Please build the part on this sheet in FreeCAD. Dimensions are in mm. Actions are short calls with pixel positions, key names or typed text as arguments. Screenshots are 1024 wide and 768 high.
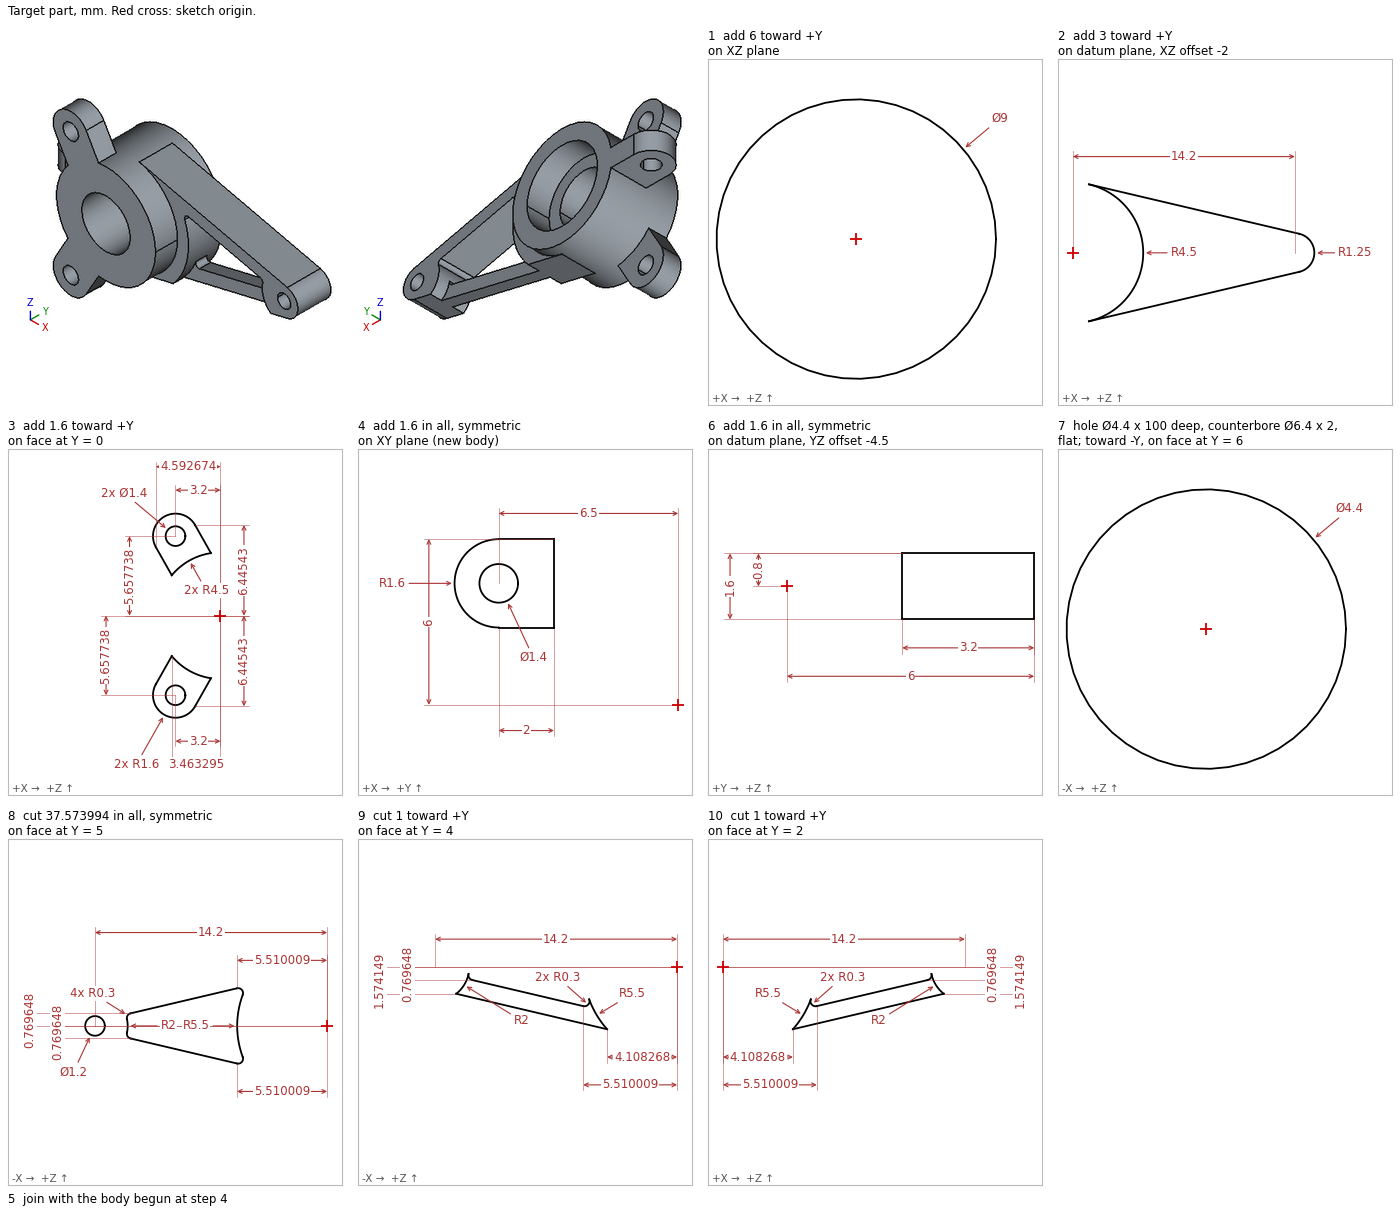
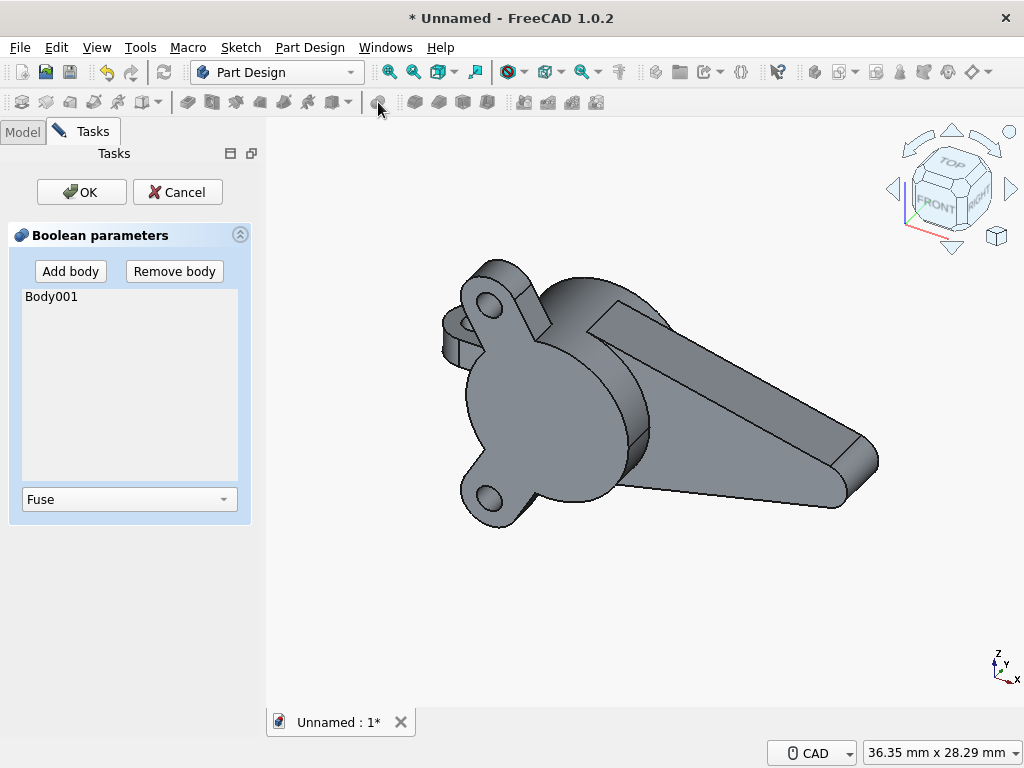
click(82, 192)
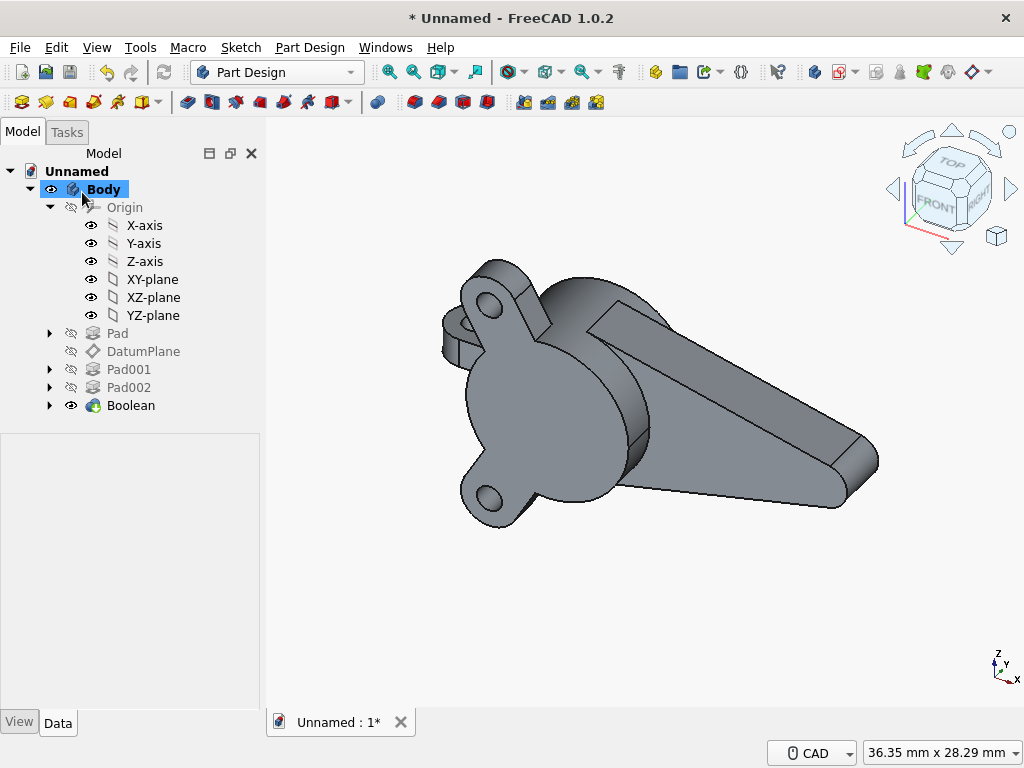
click(136, 315)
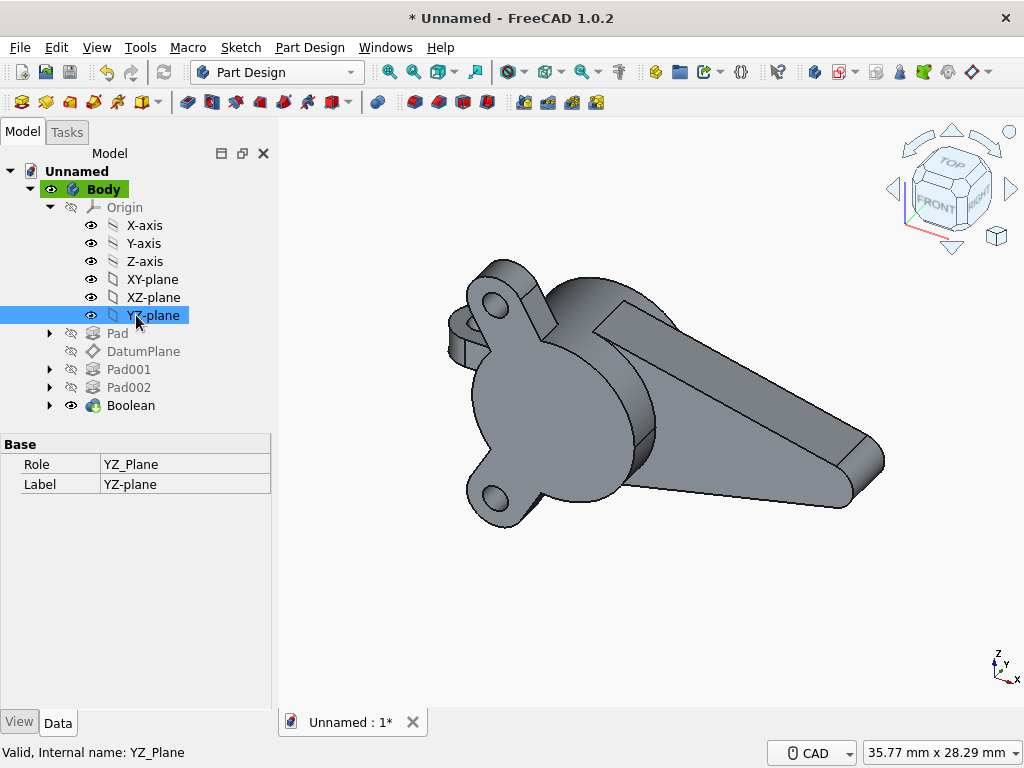
click(972, 72)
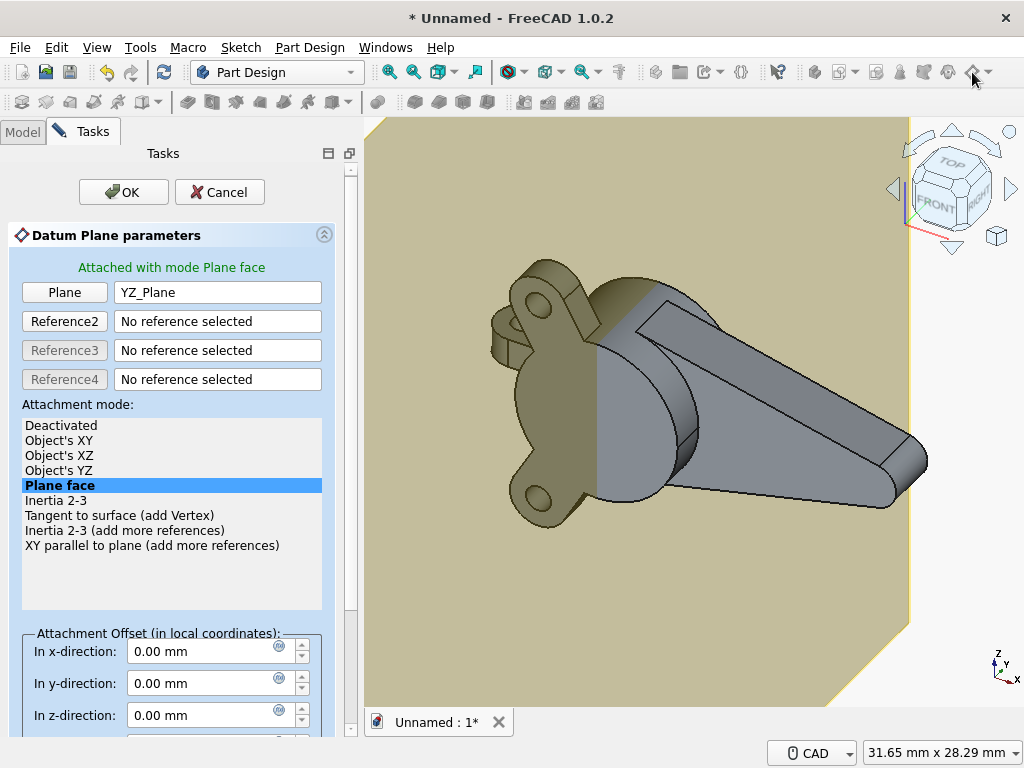
triple_click(210, 715)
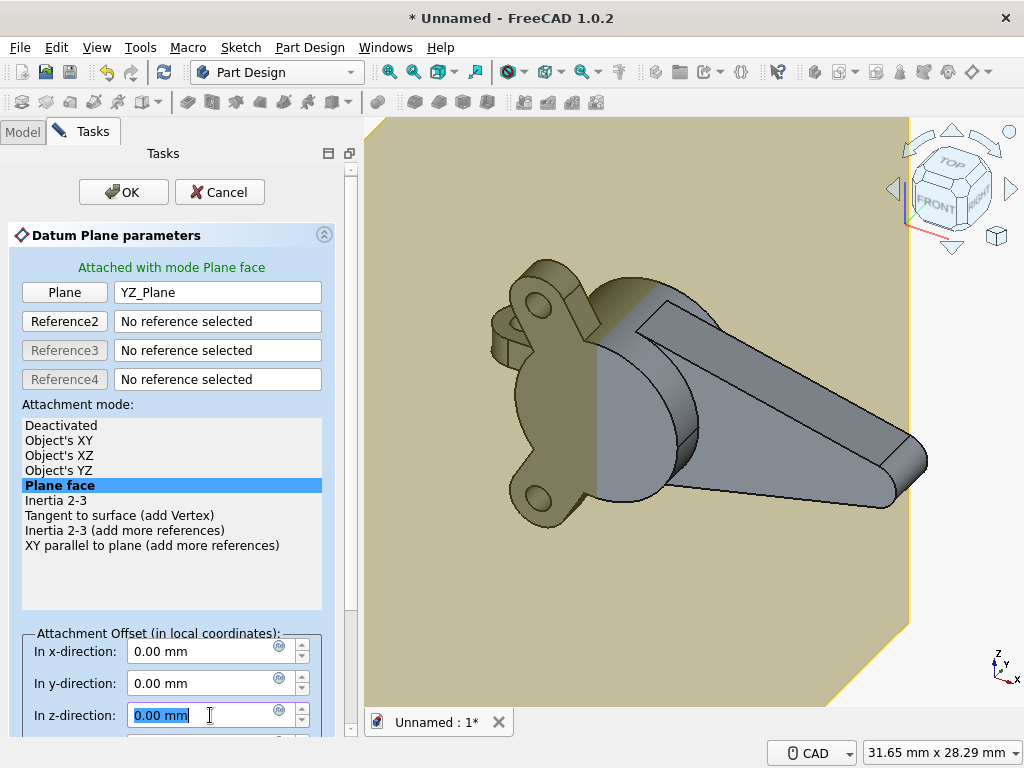
text(-4.5)
key(Tab)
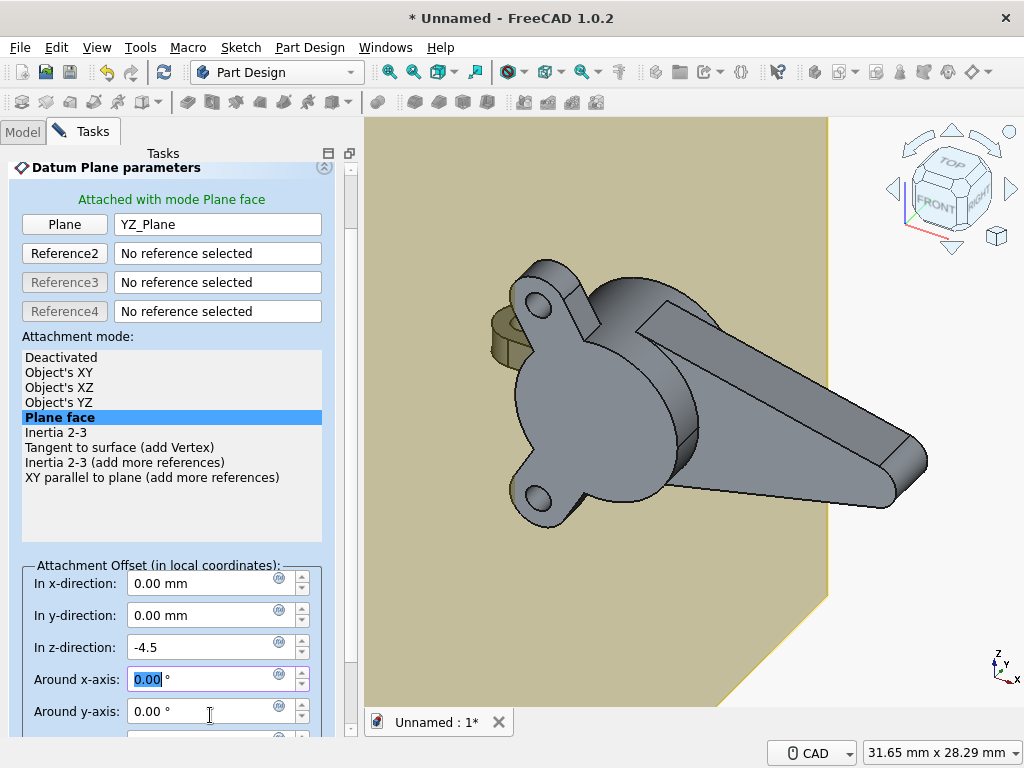
scroll(351, 450, up, 2)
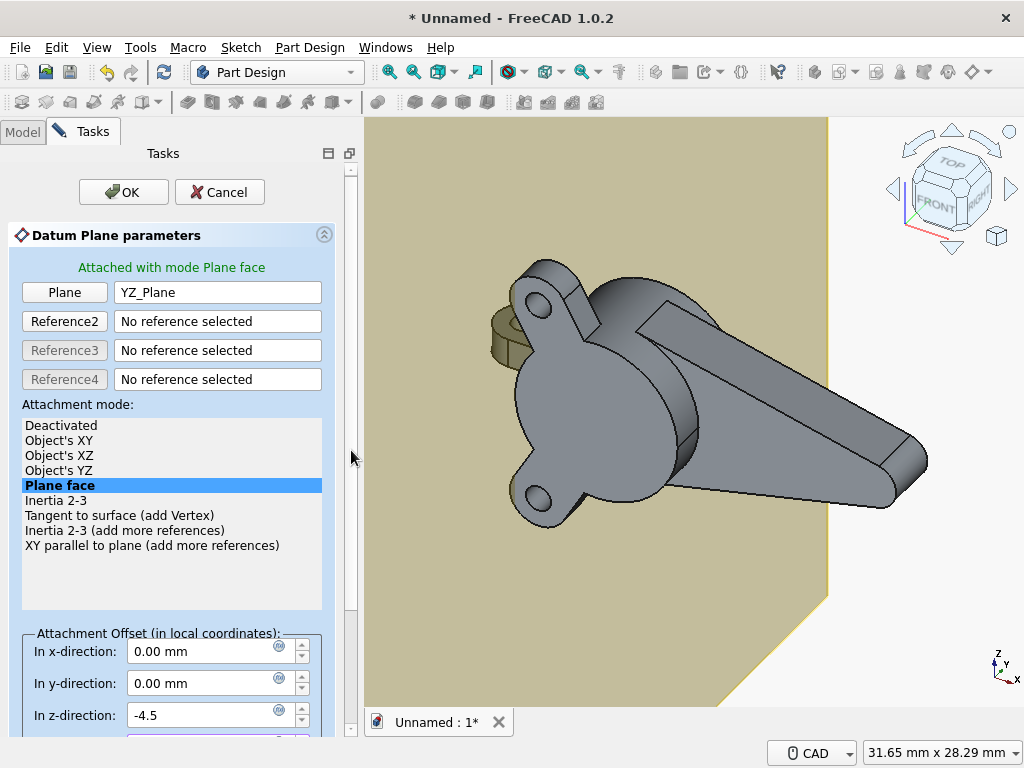
click(124, 192)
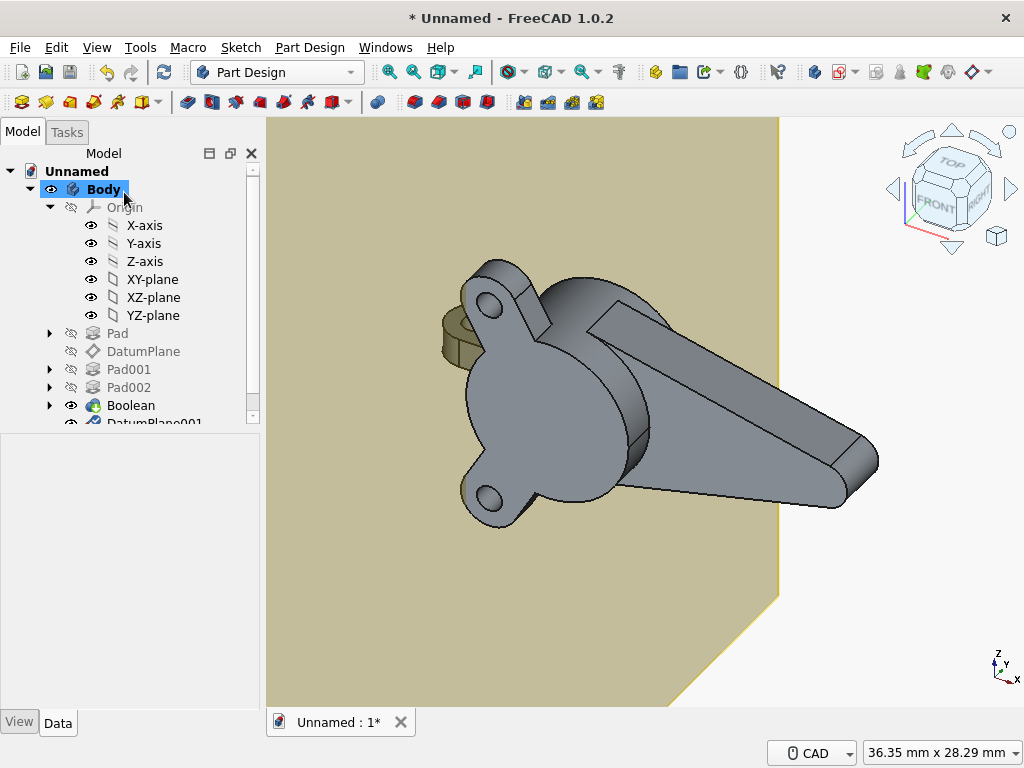
click(116, 423)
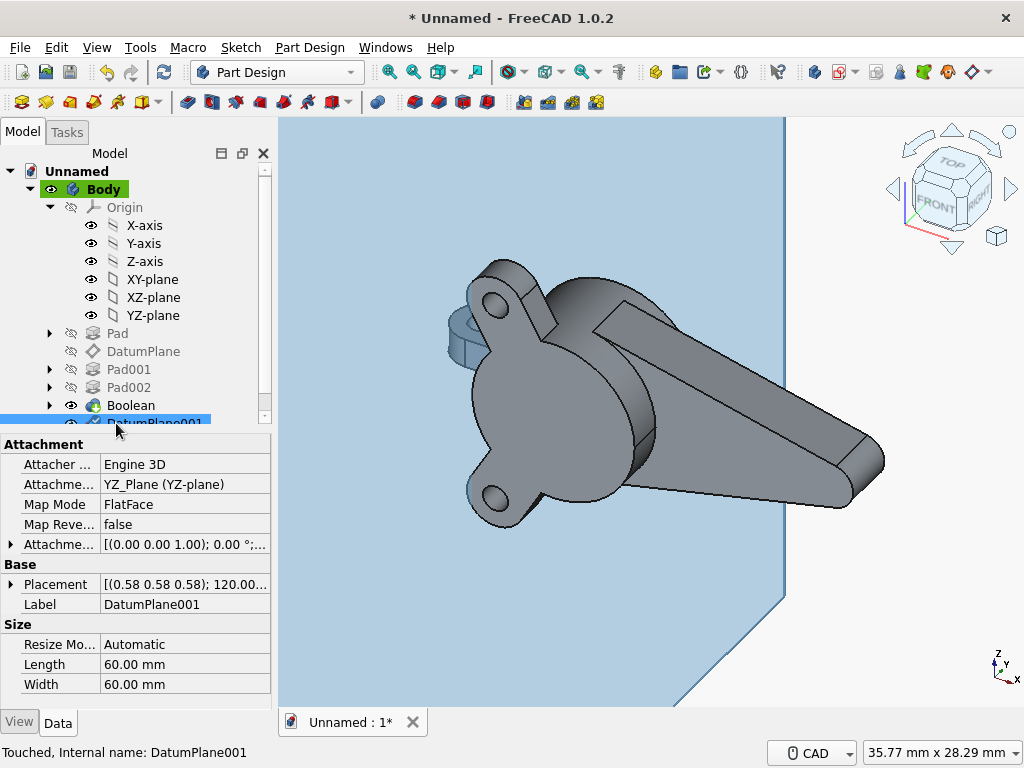
click(840, 72)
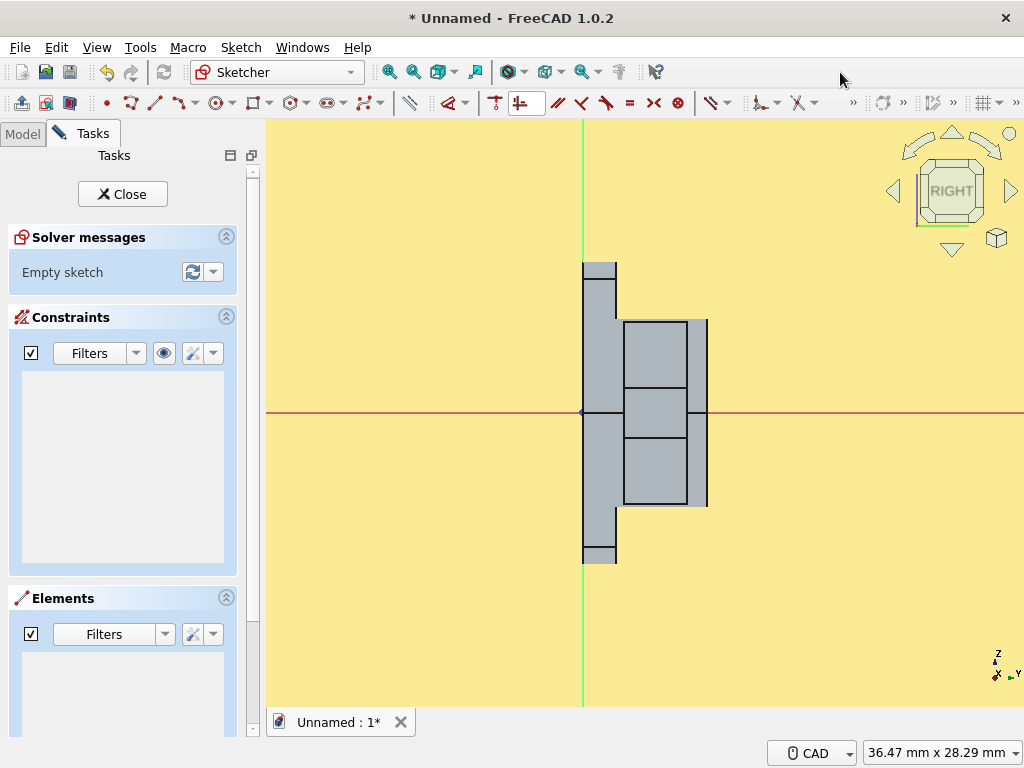
click(70, 104)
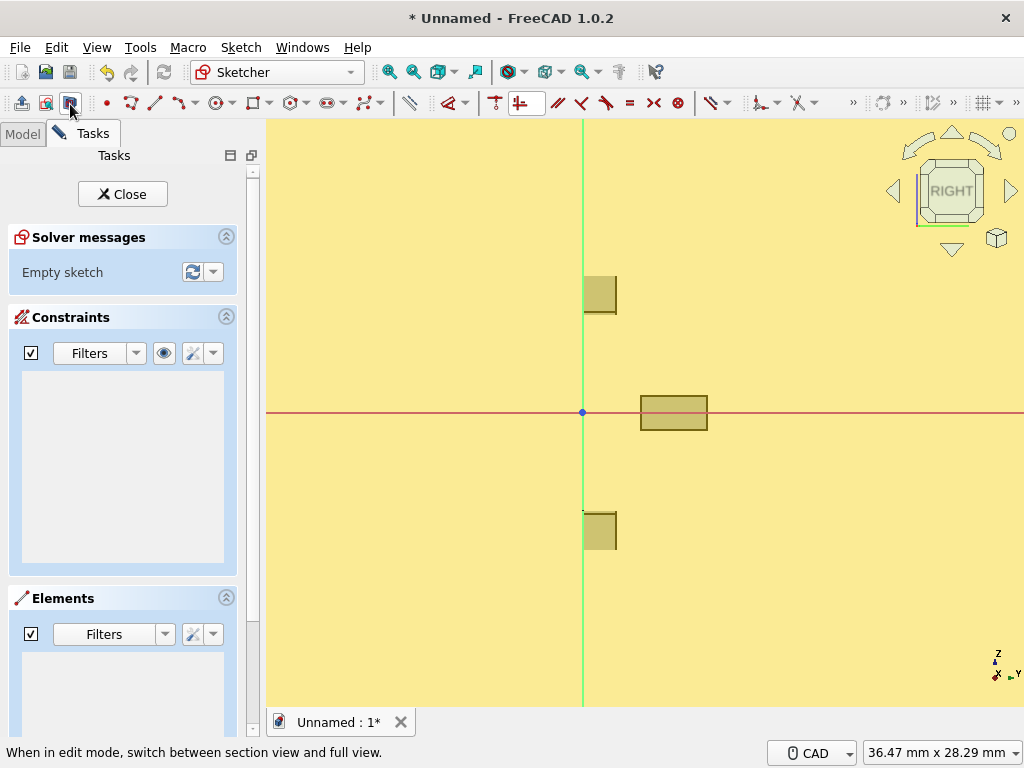
scroll(675, 413, up, 6)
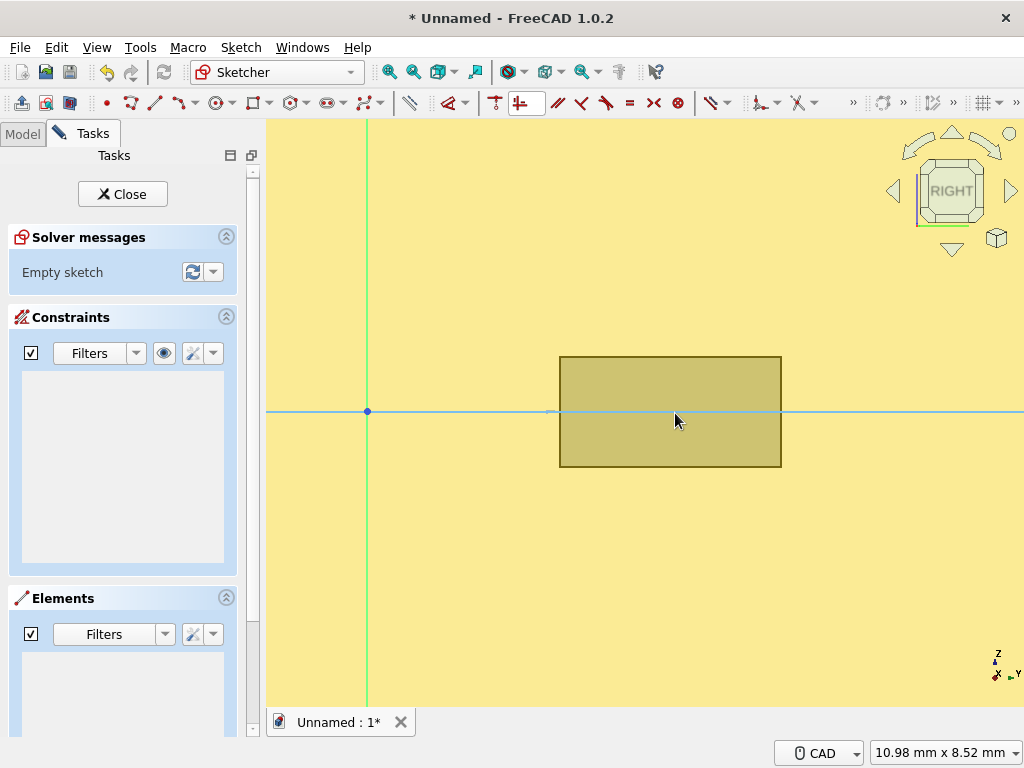
click(254, 104)